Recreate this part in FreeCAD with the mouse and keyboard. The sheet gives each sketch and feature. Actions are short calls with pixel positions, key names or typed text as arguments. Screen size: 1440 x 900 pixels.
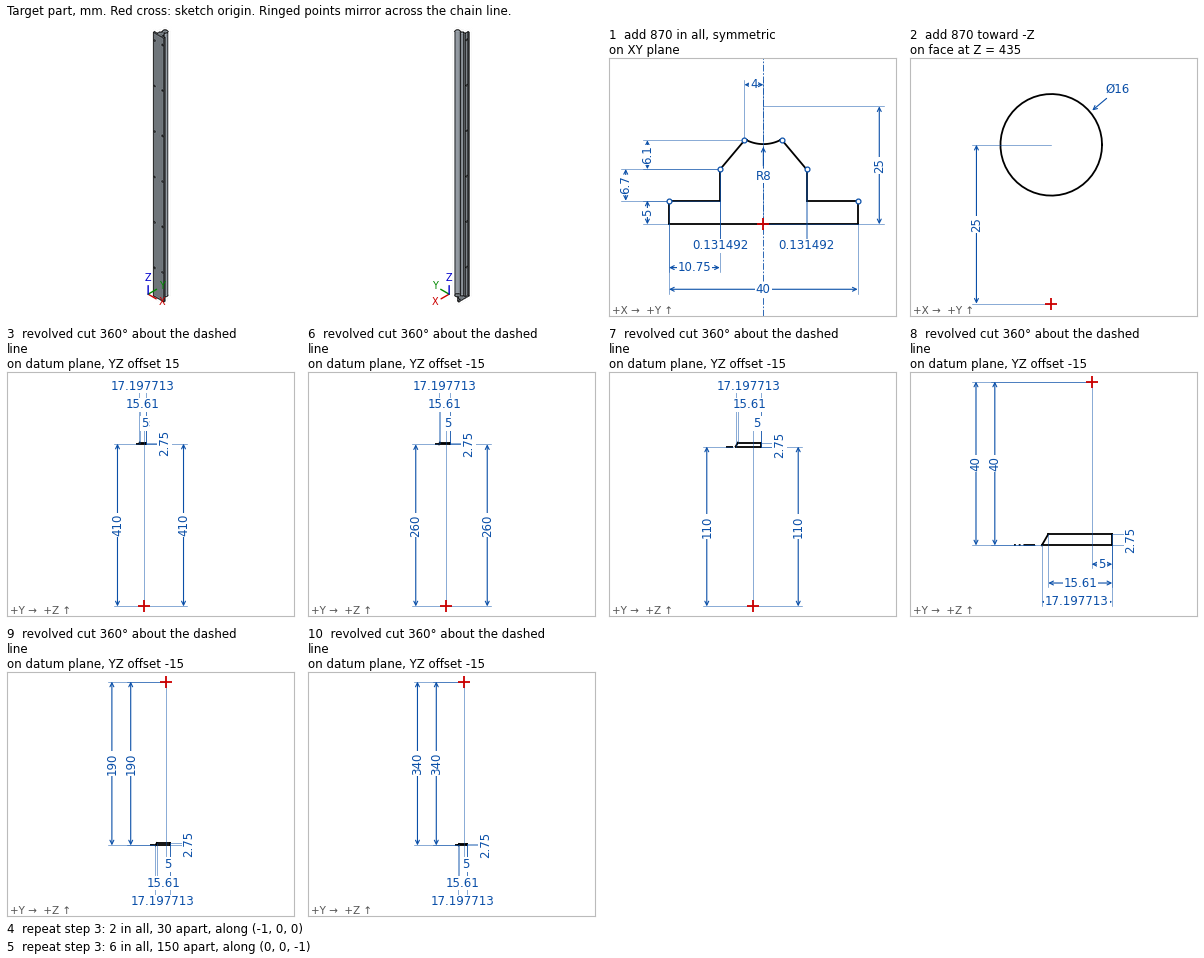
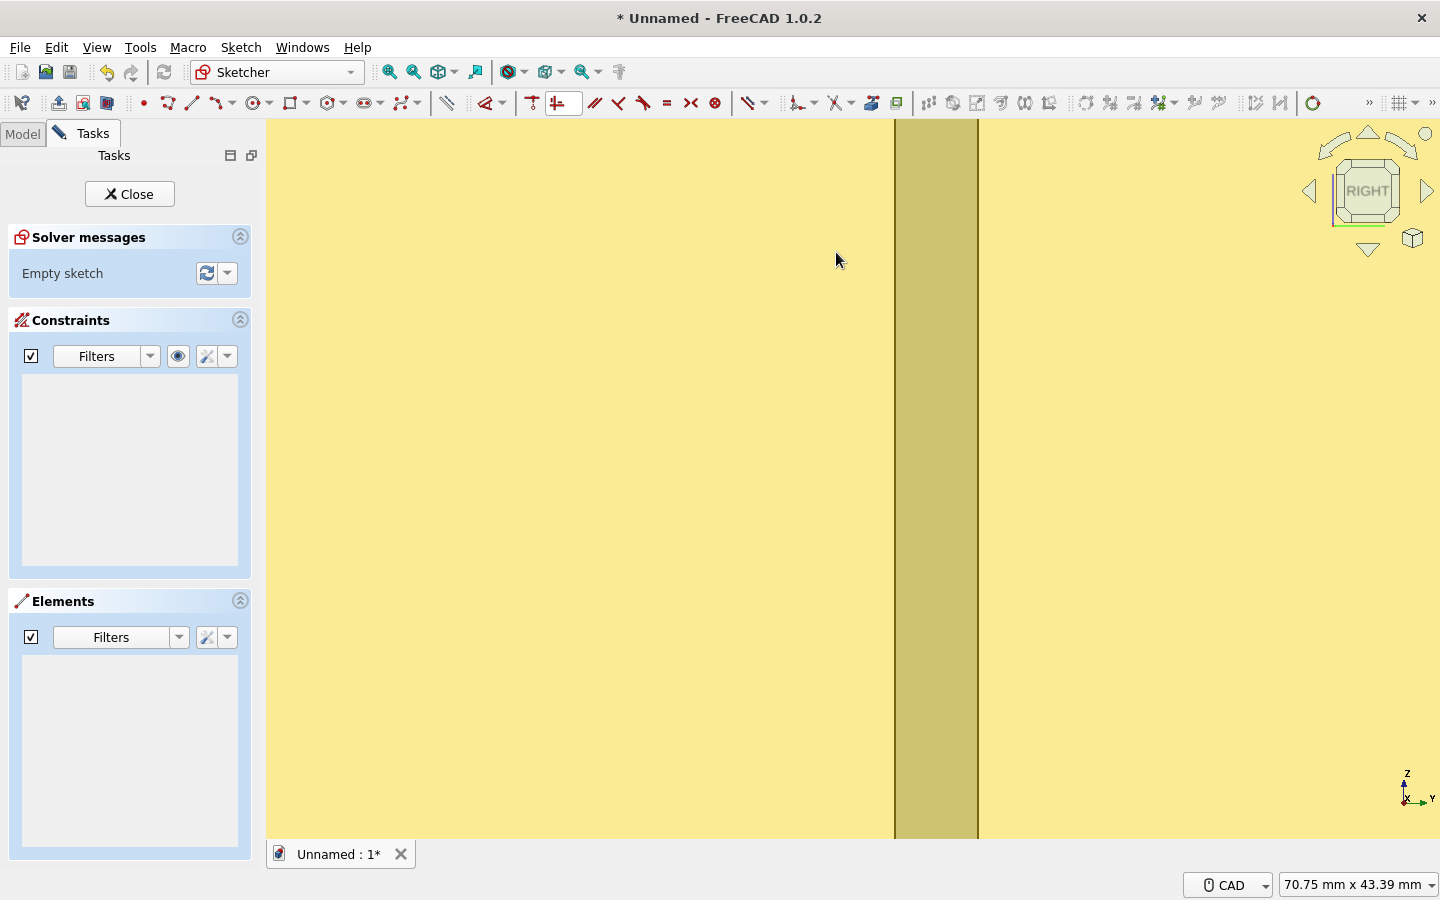
scroll(770, 461, up, 3)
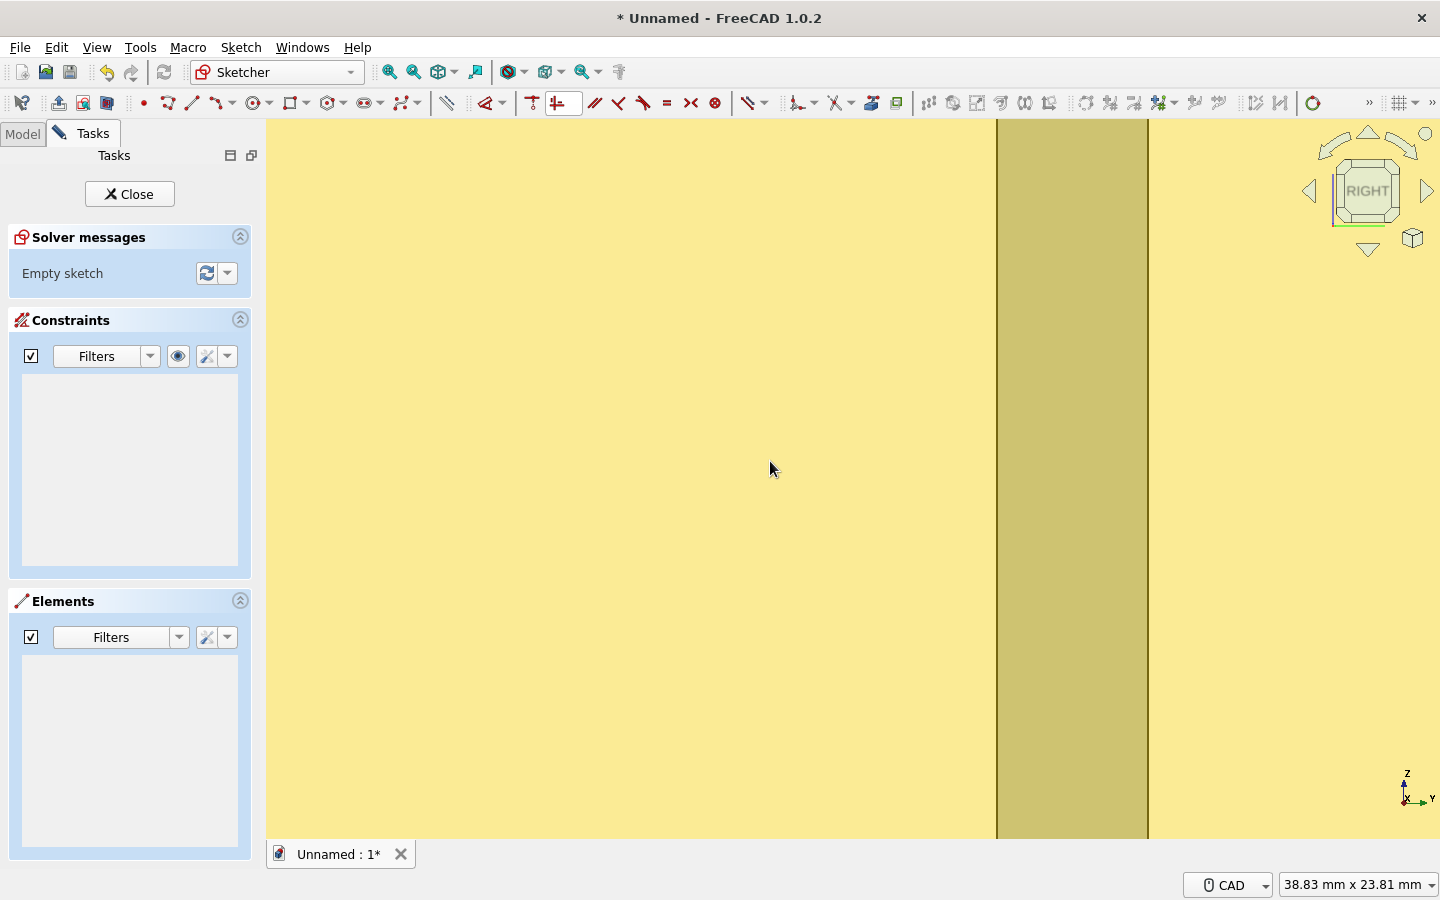
click(168, 104)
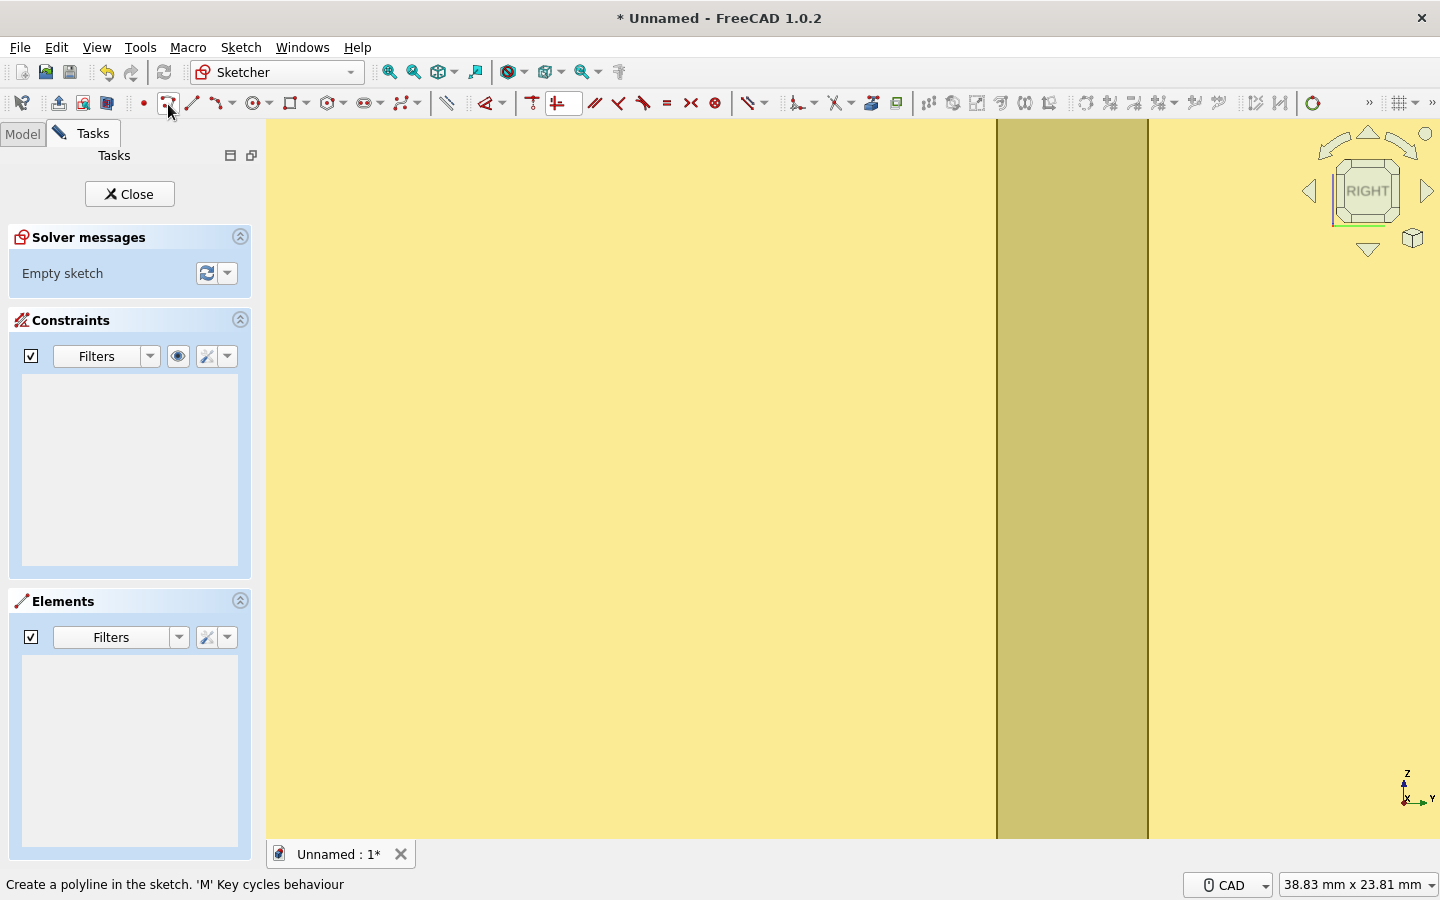
click(1148, 520)
click(1148, 437)
click(676, 437)
click(628, 520)
click(1148, 521)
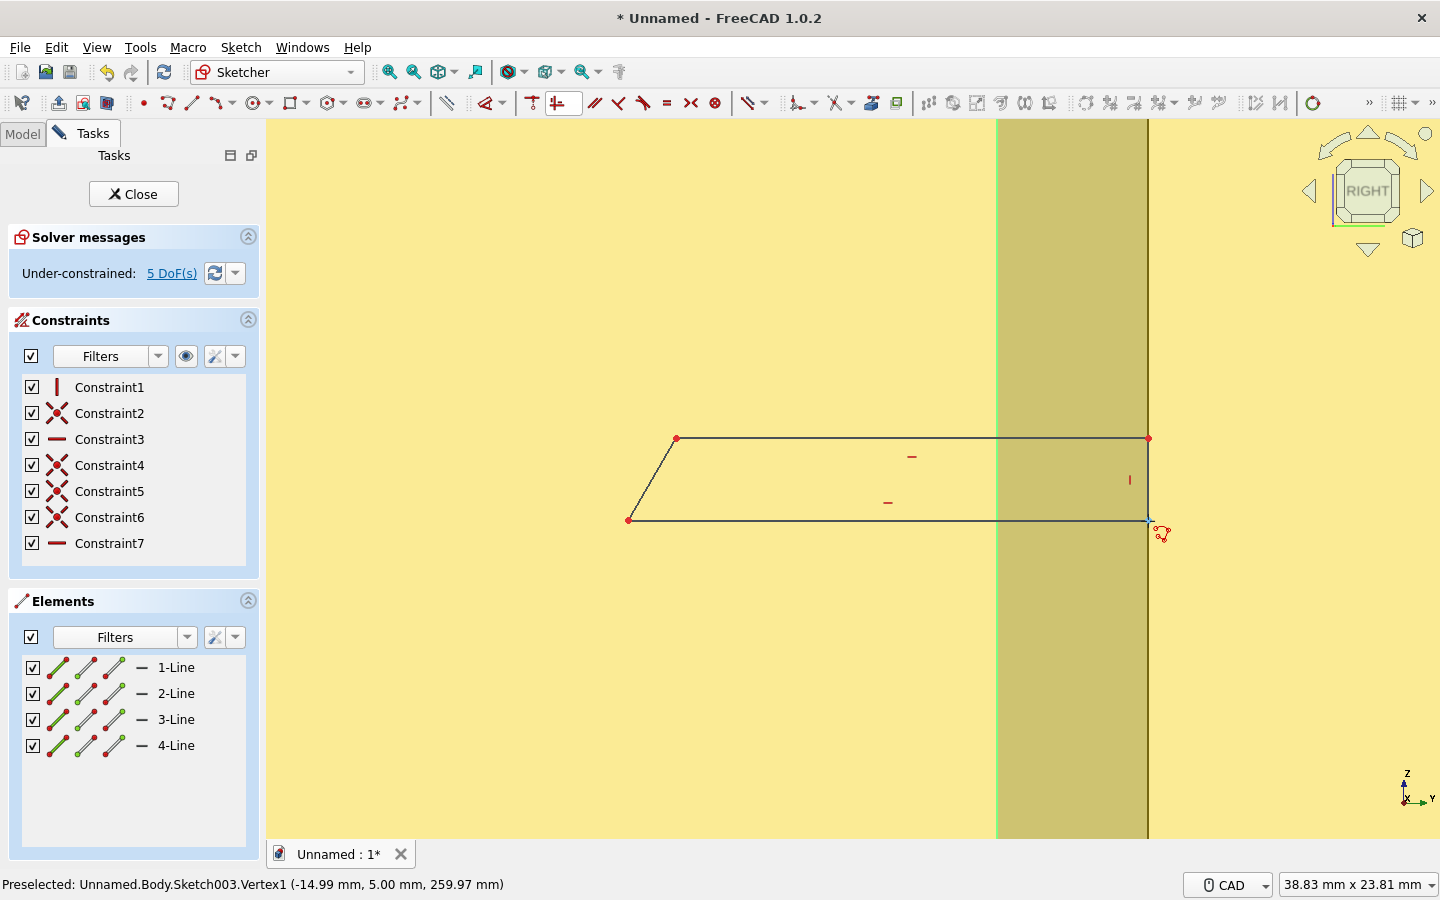
key(g)
key(l)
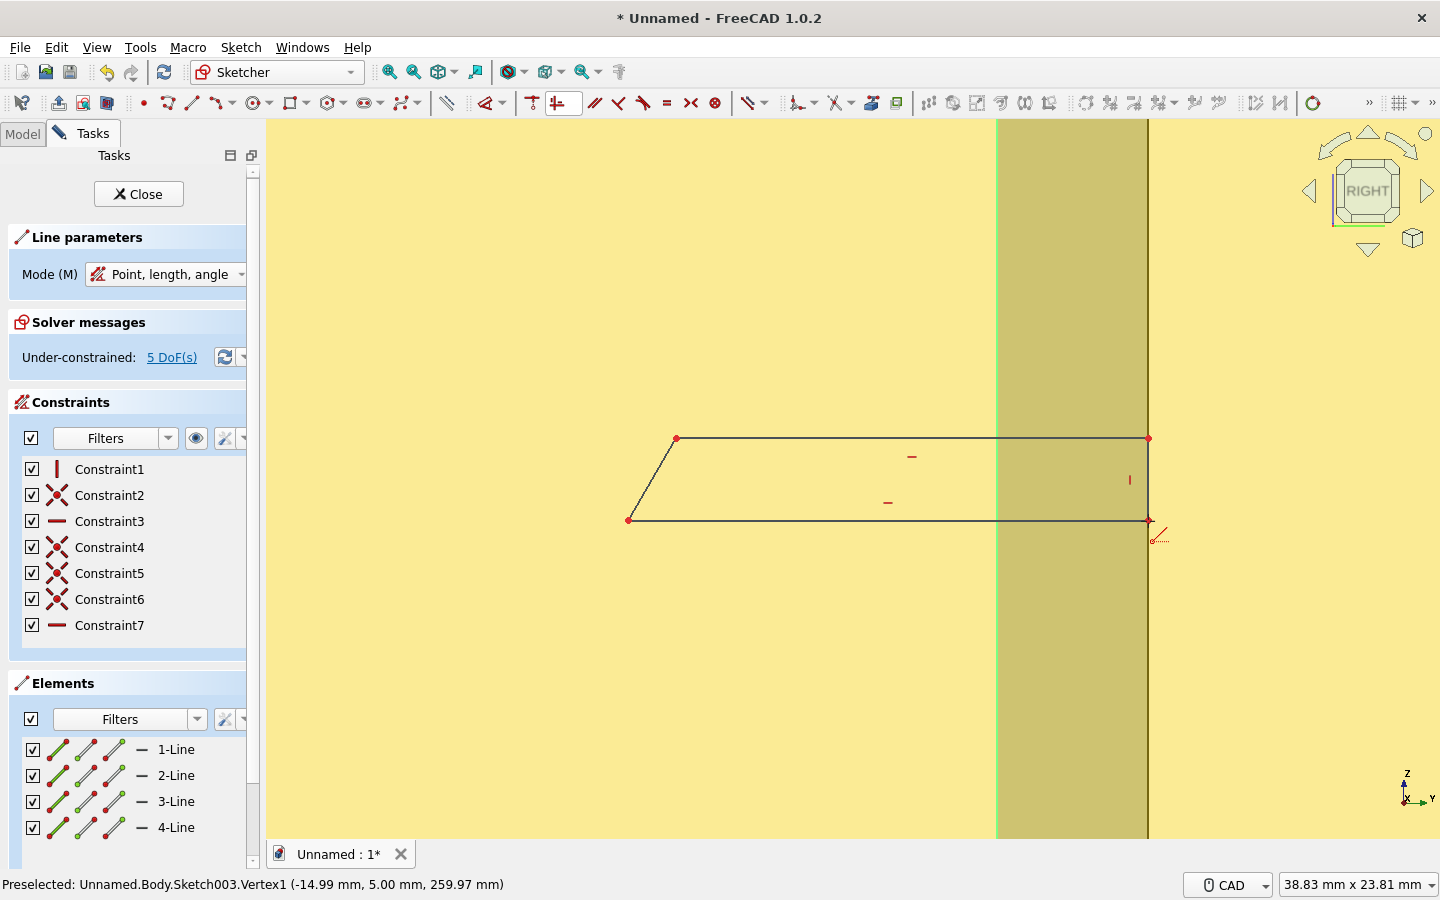
click(576, 520)
click(420, 520)
key(Escape)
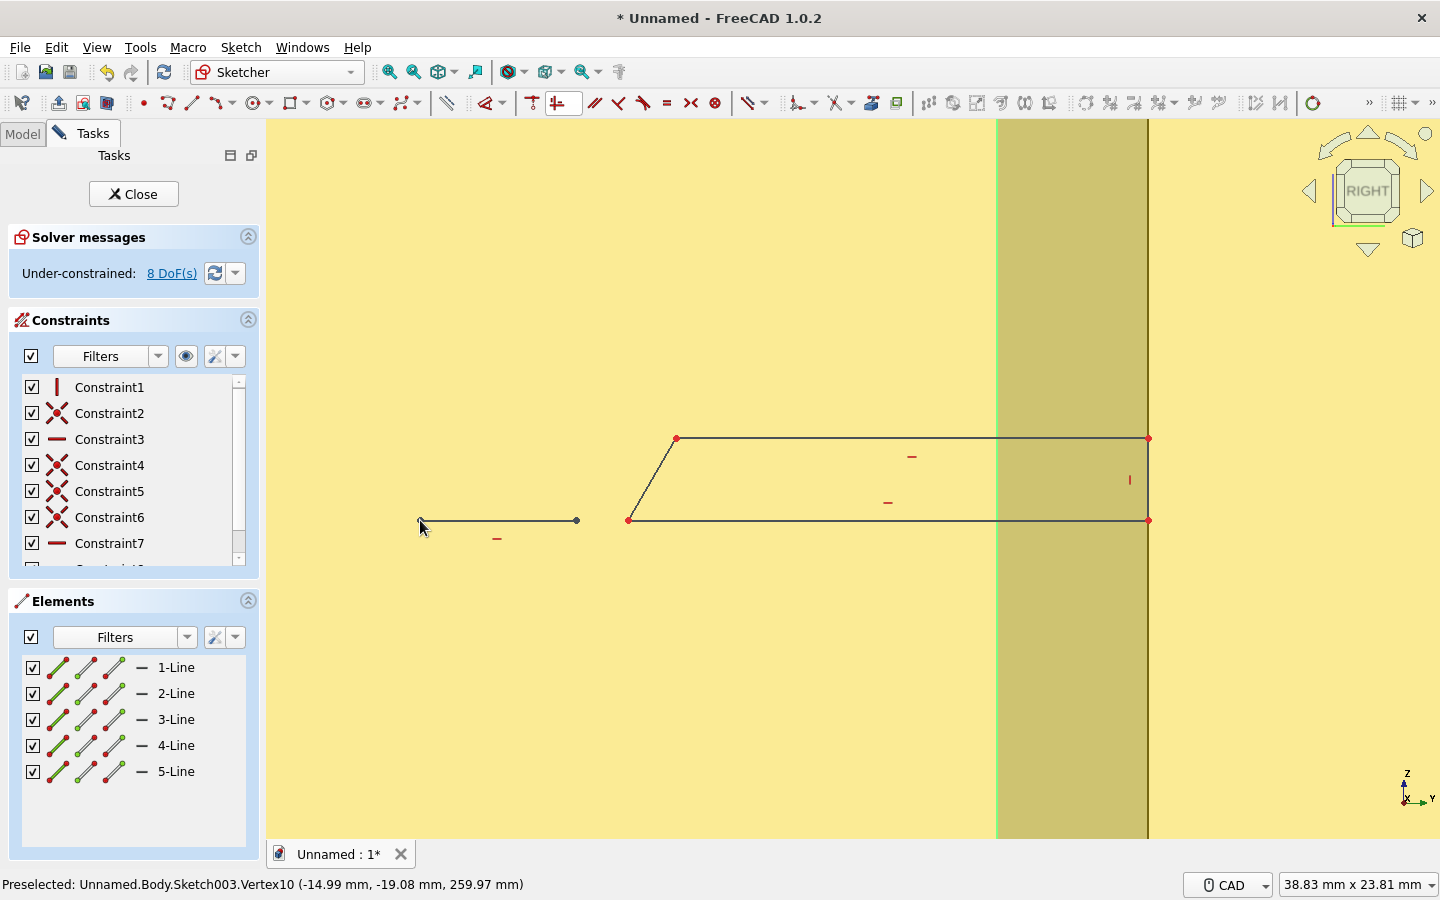
click(529, 521)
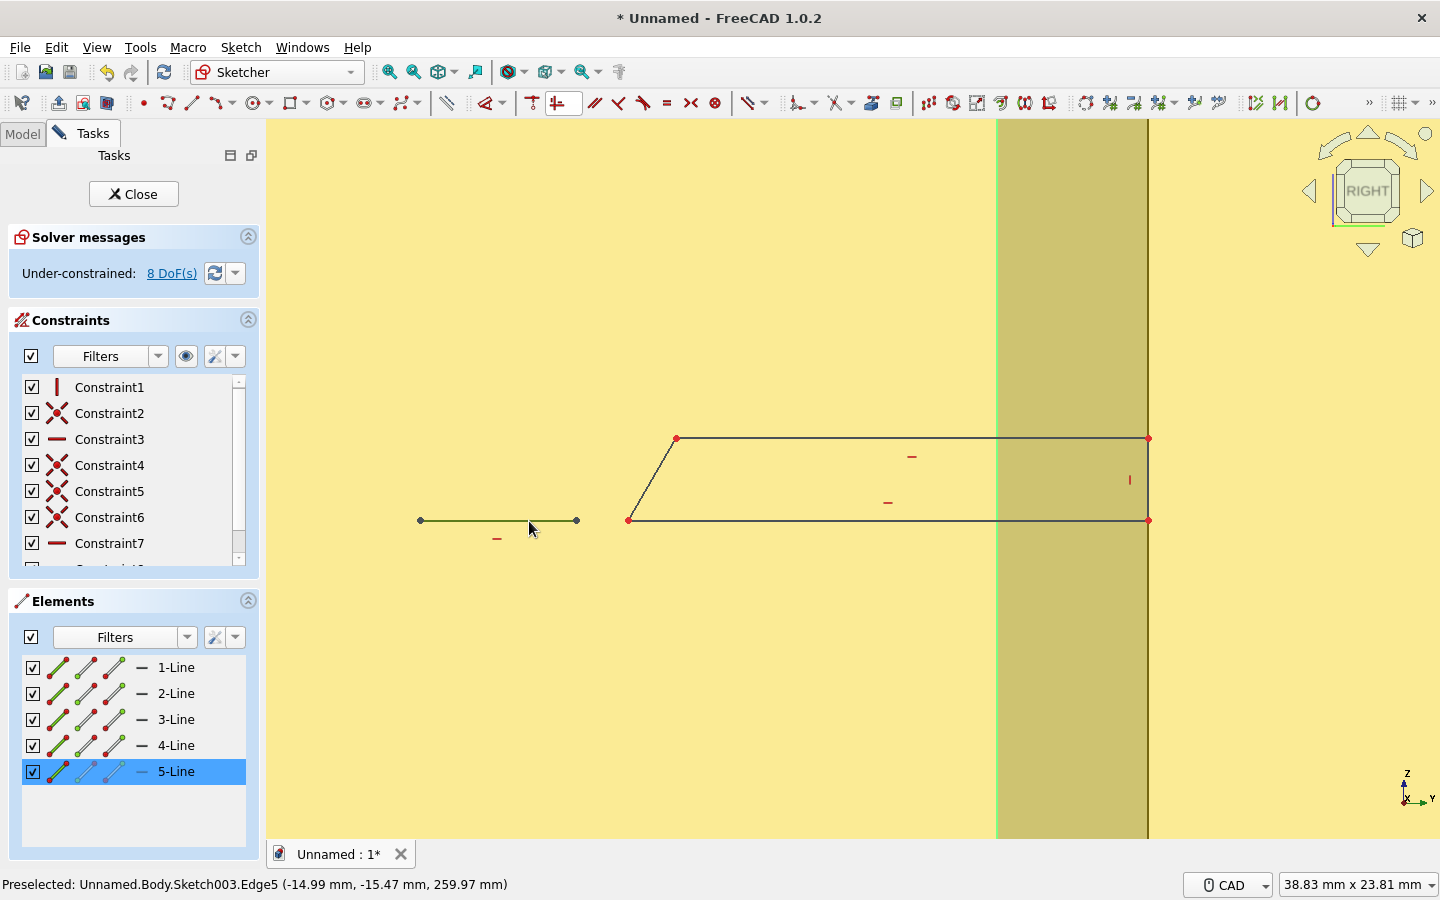
click(448, 104)